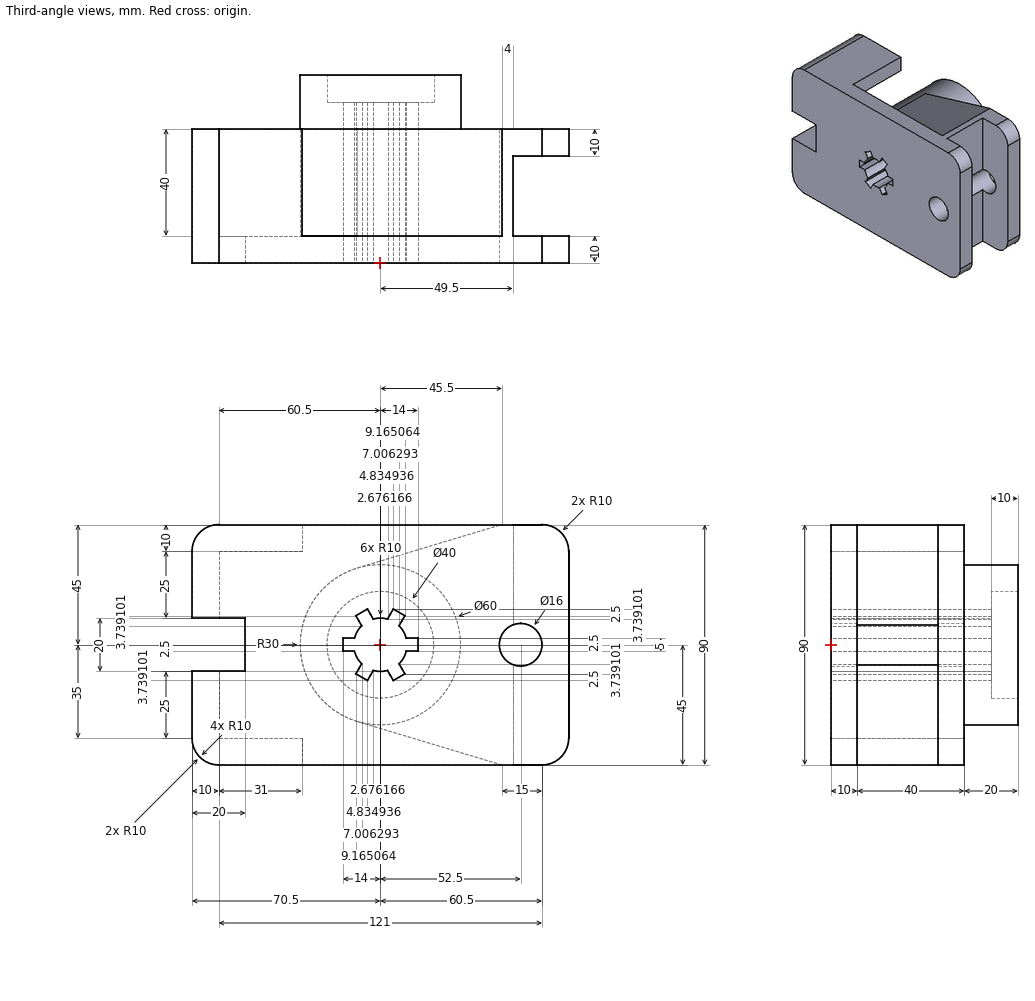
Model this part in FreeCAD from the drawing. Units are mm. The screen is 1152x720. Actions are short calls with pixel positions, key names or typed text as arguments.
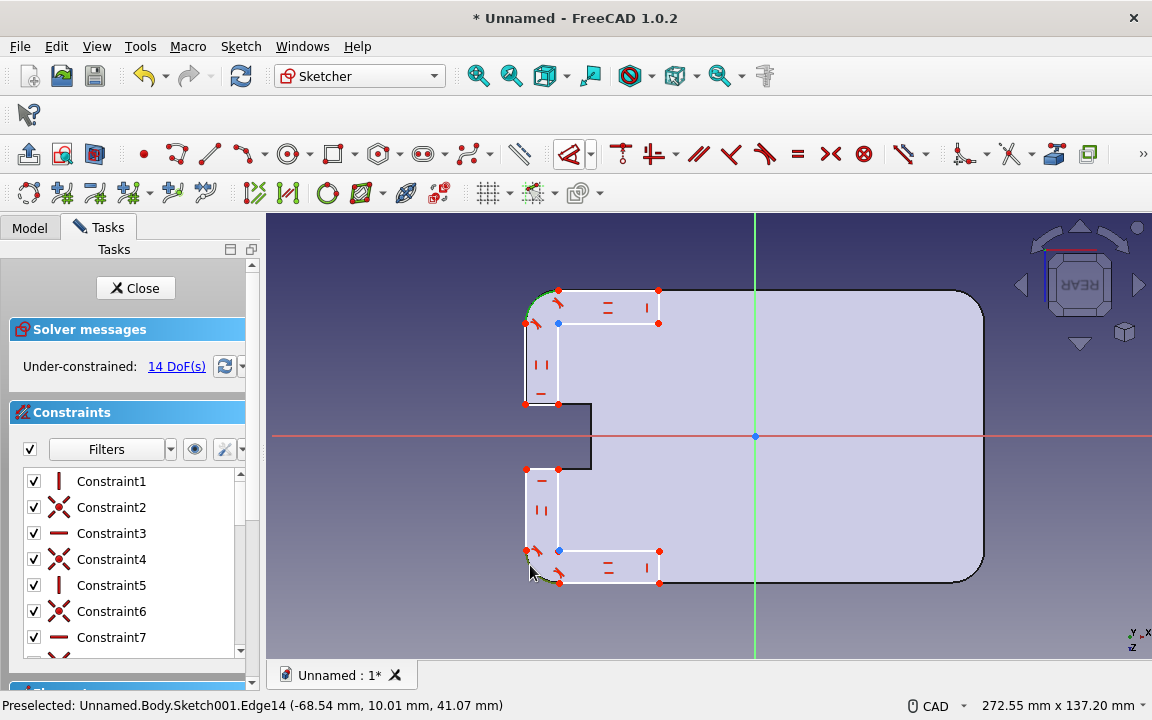
click(798, 154)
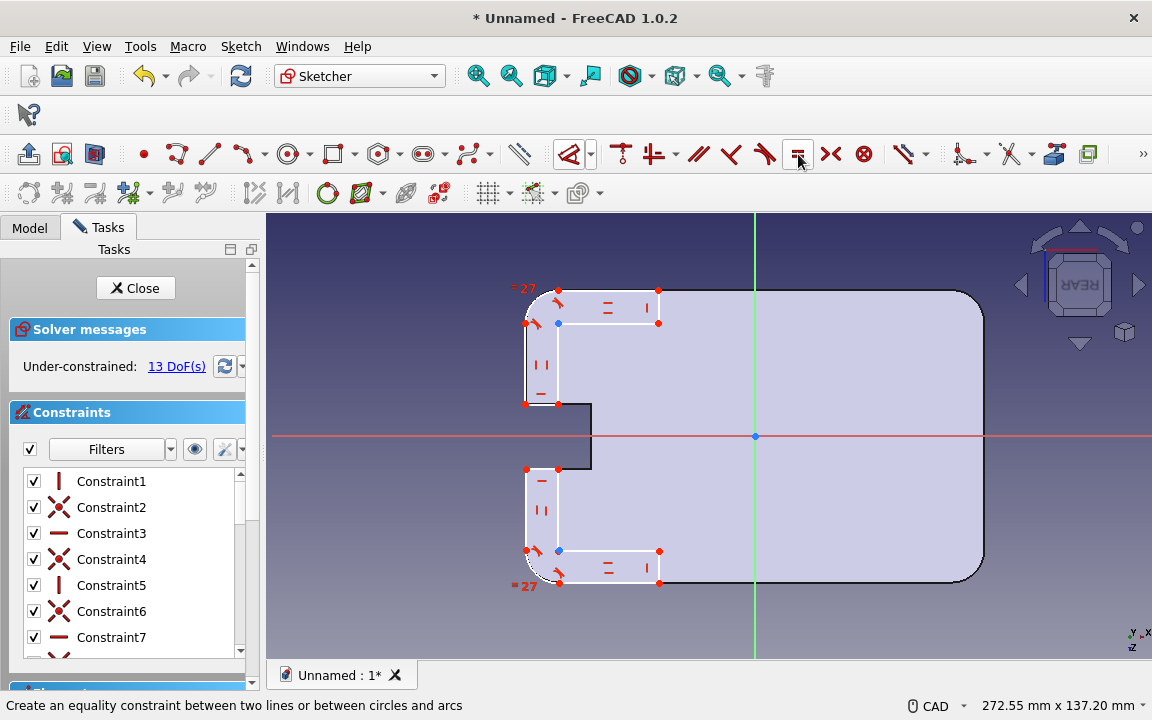
click(543, 295)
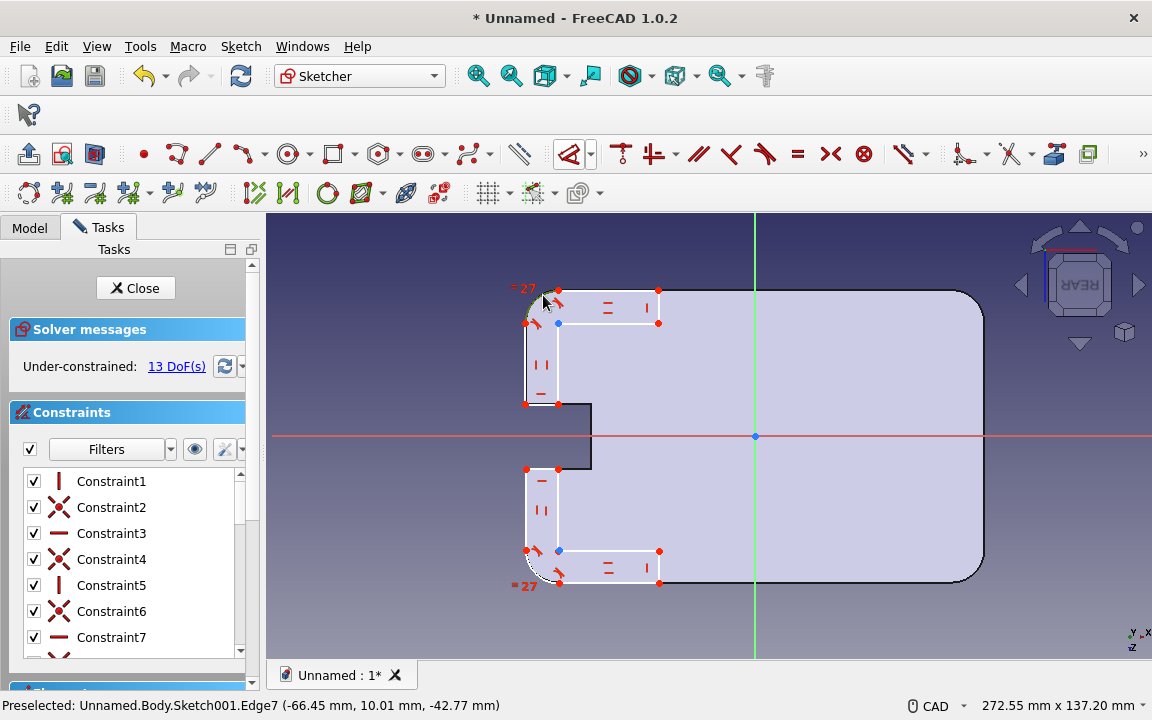
click(590, 154)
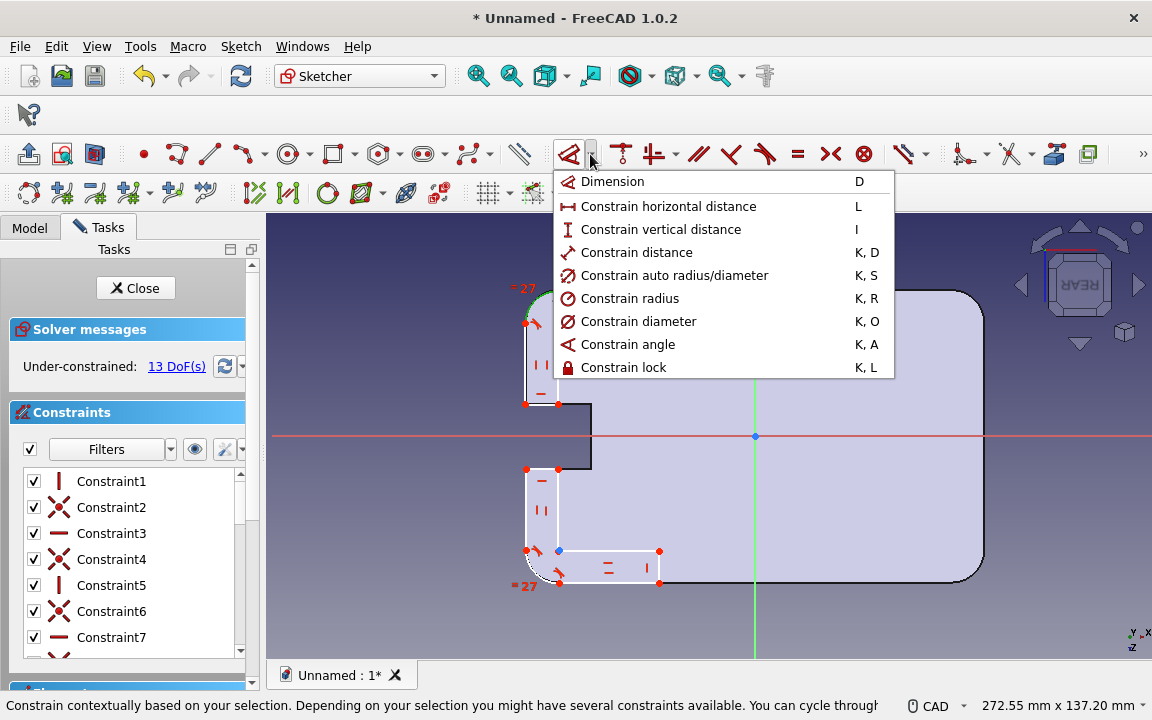
click(724, 298)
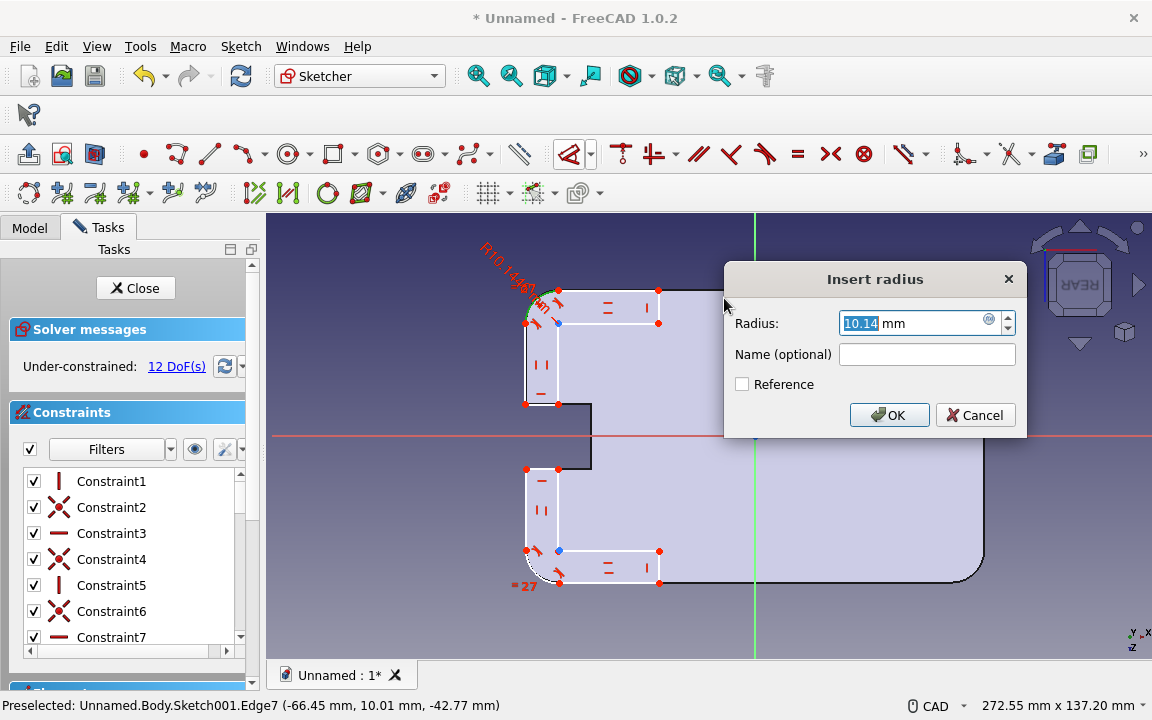
text(10)
key(Return)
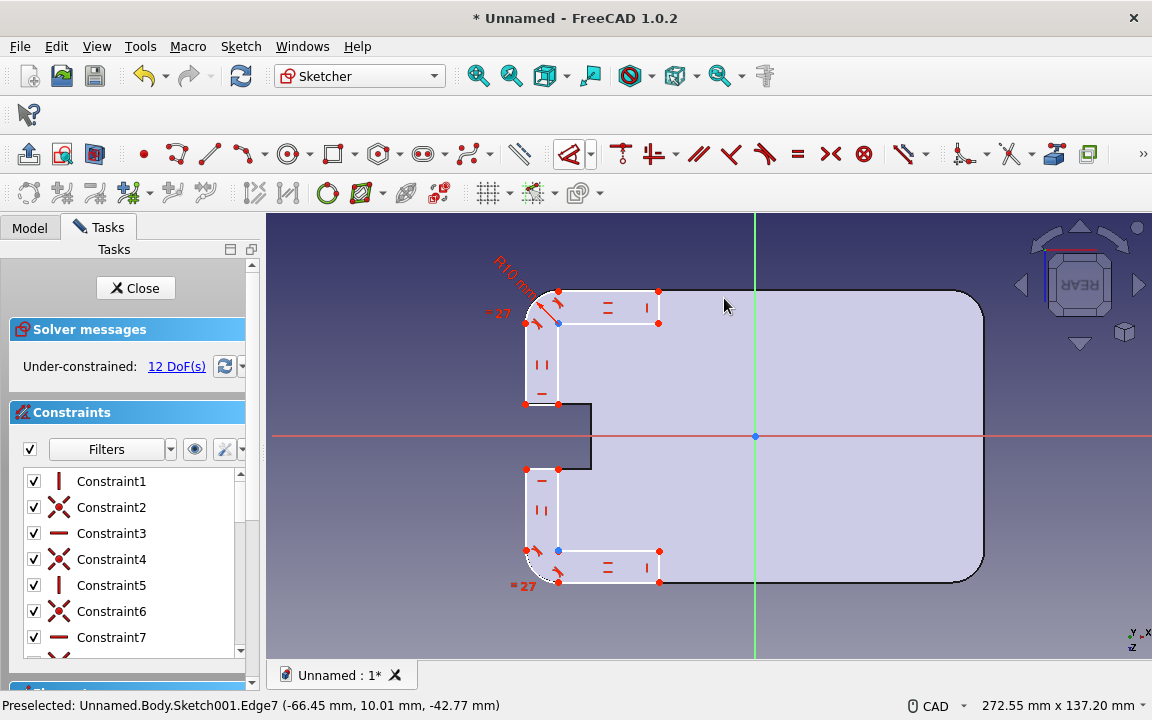
click(526, 348)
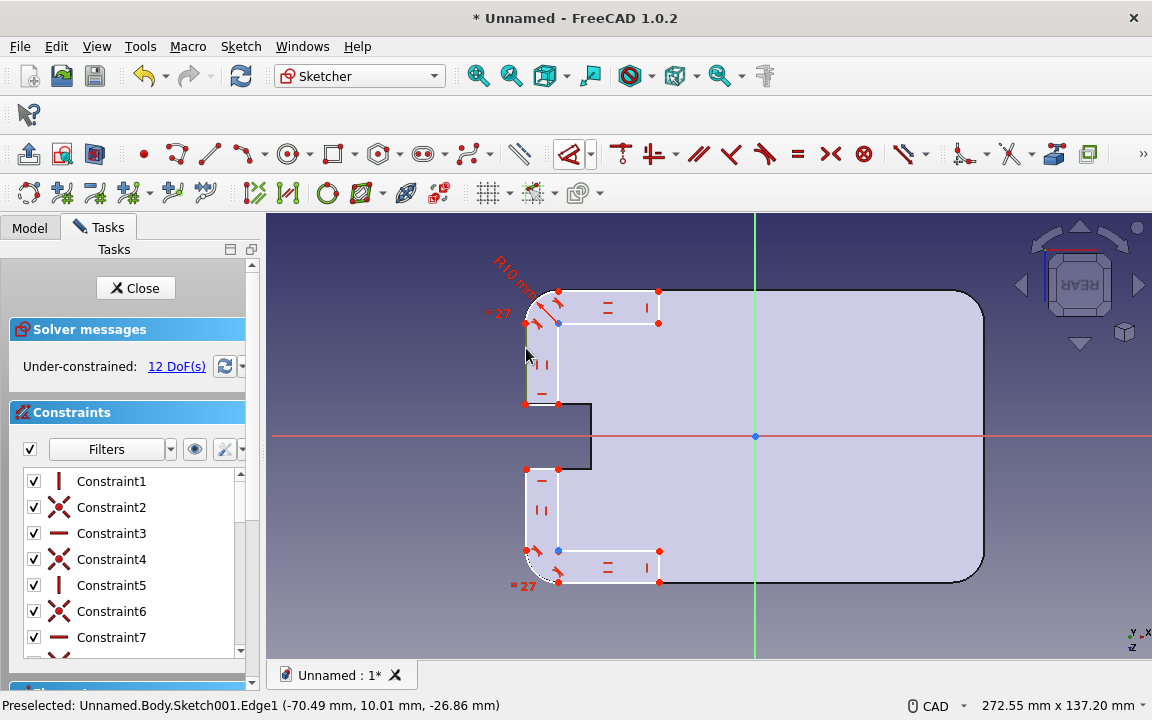
key(i)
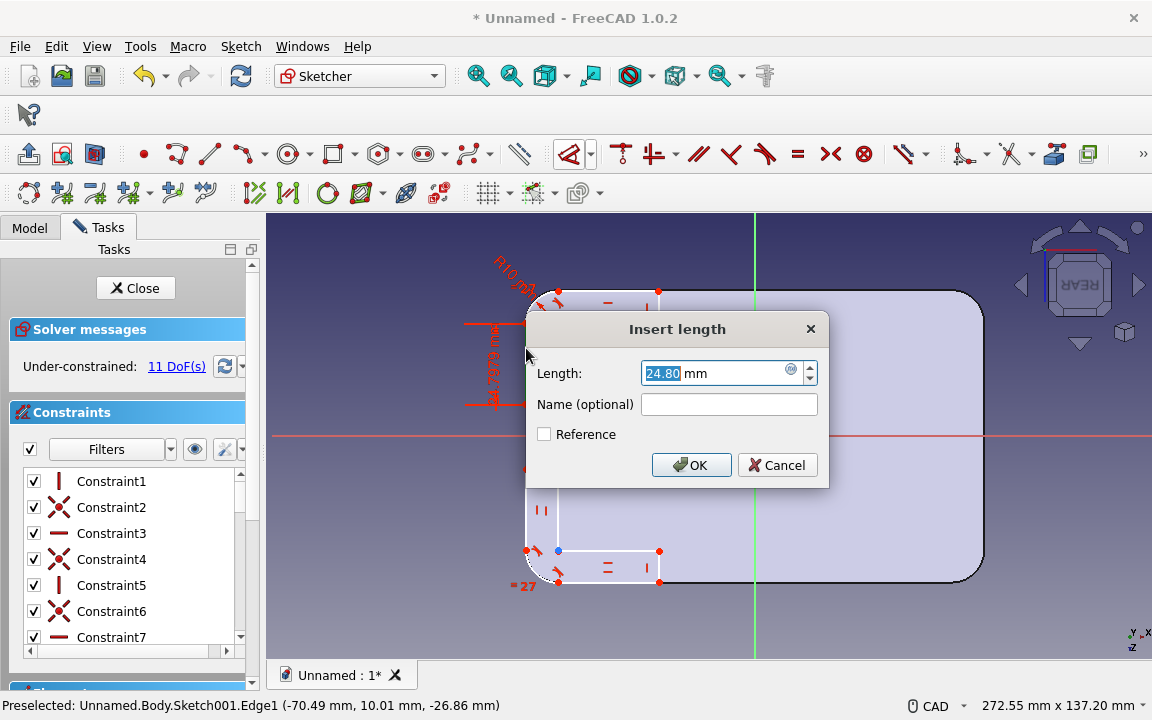
text(25)
key(Return)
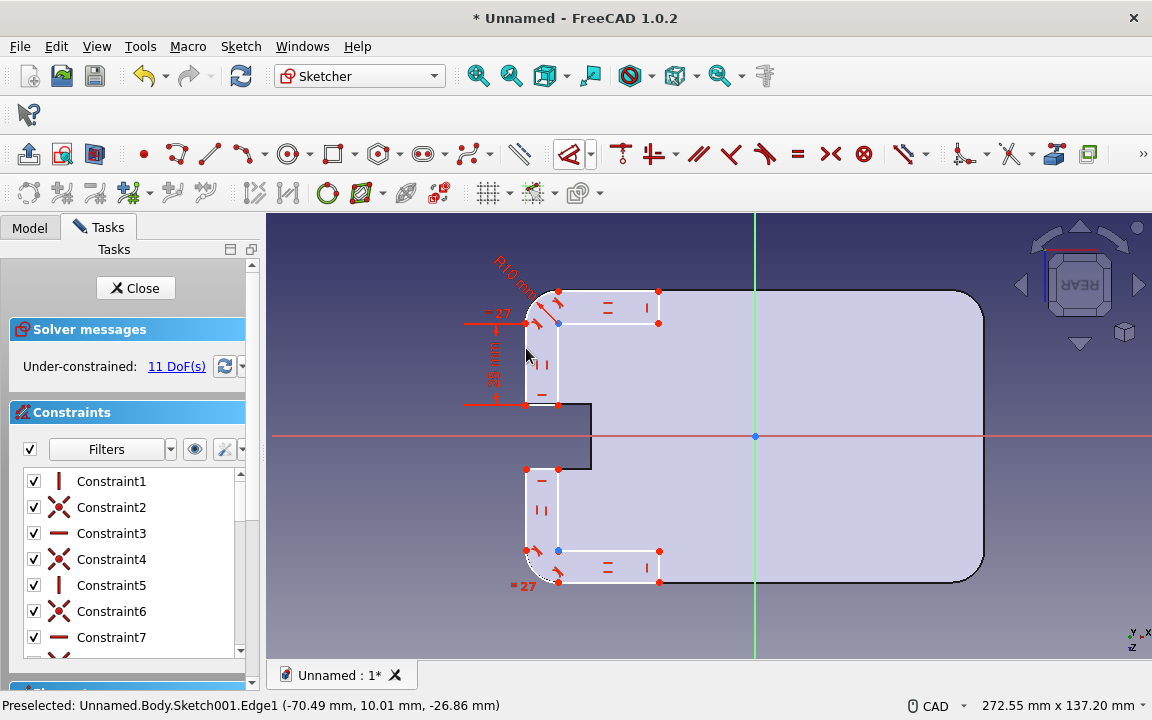
scroll(536, 405, up, 2)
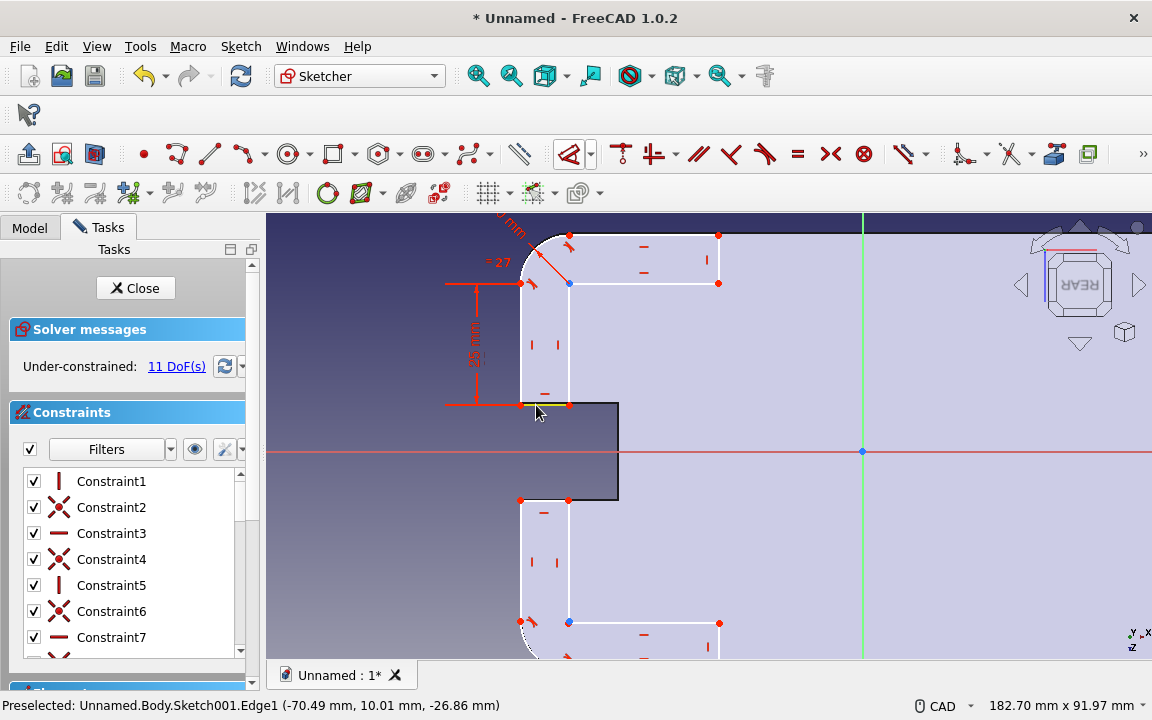
click(535, 405)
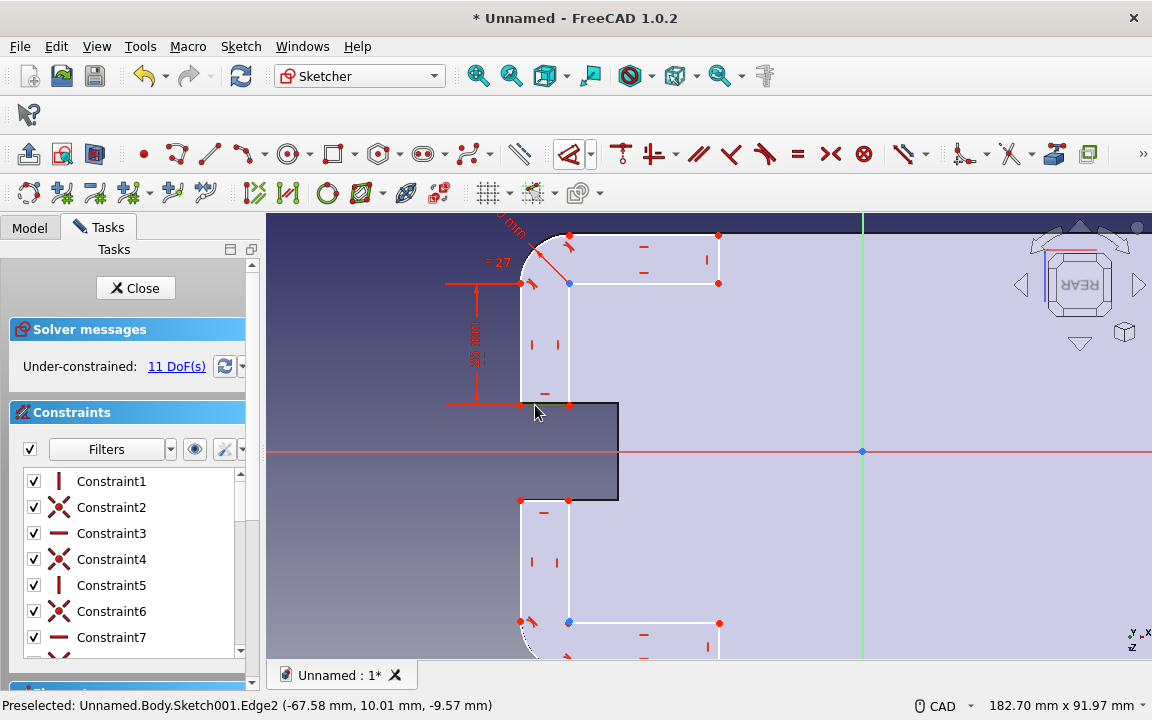
key(l)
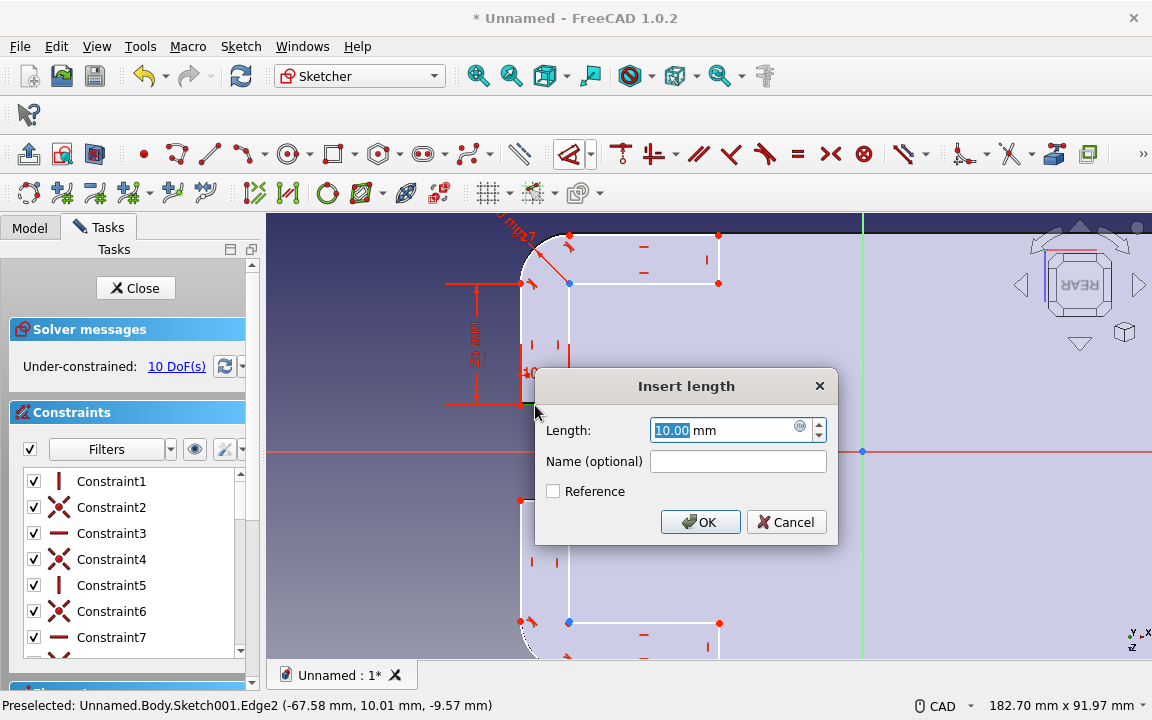
text(10)
key(Return)